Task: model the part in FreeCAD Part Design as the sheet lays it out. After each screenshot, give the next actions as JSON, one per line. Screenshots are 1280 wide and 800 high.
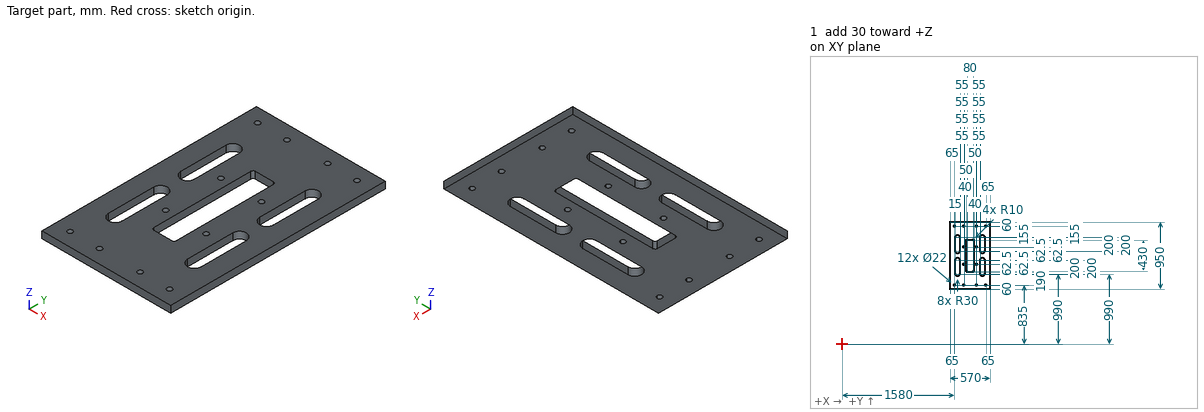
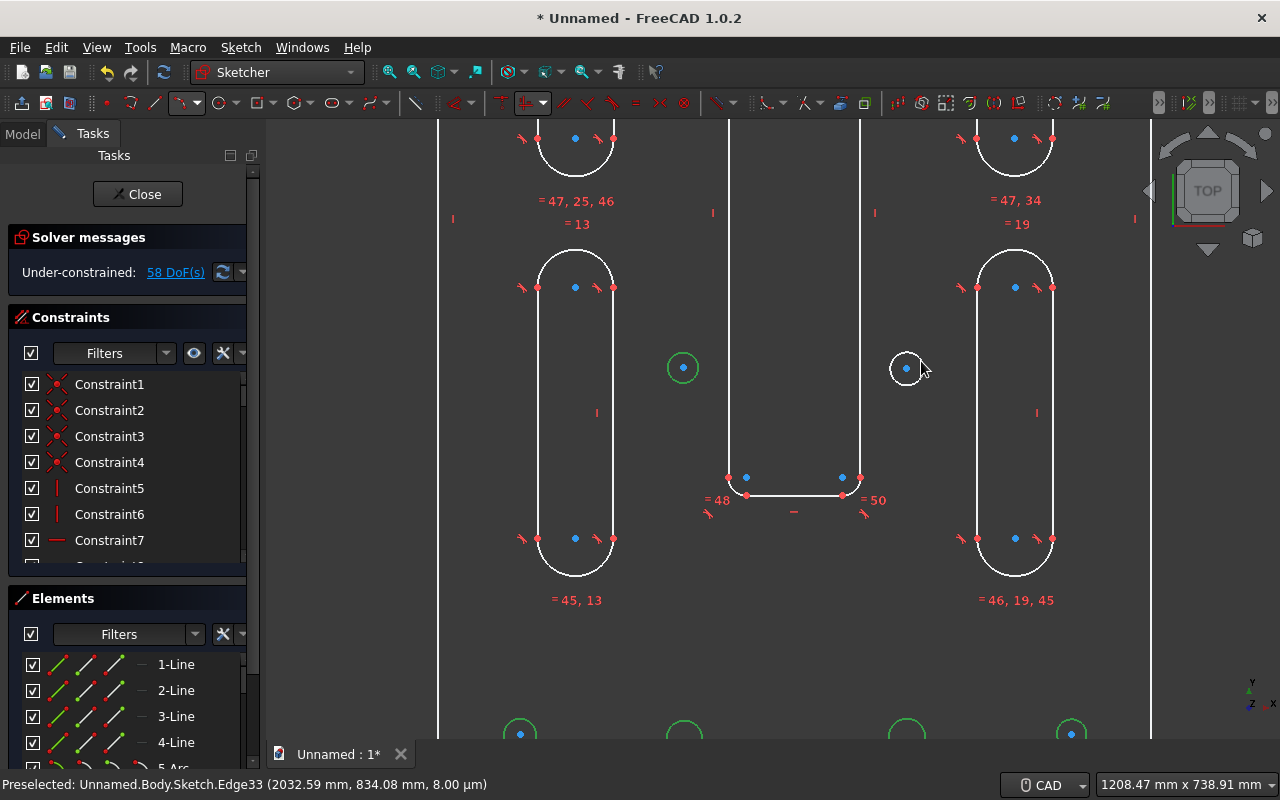
{"action": "left_click", "coordinate": [919, 357]}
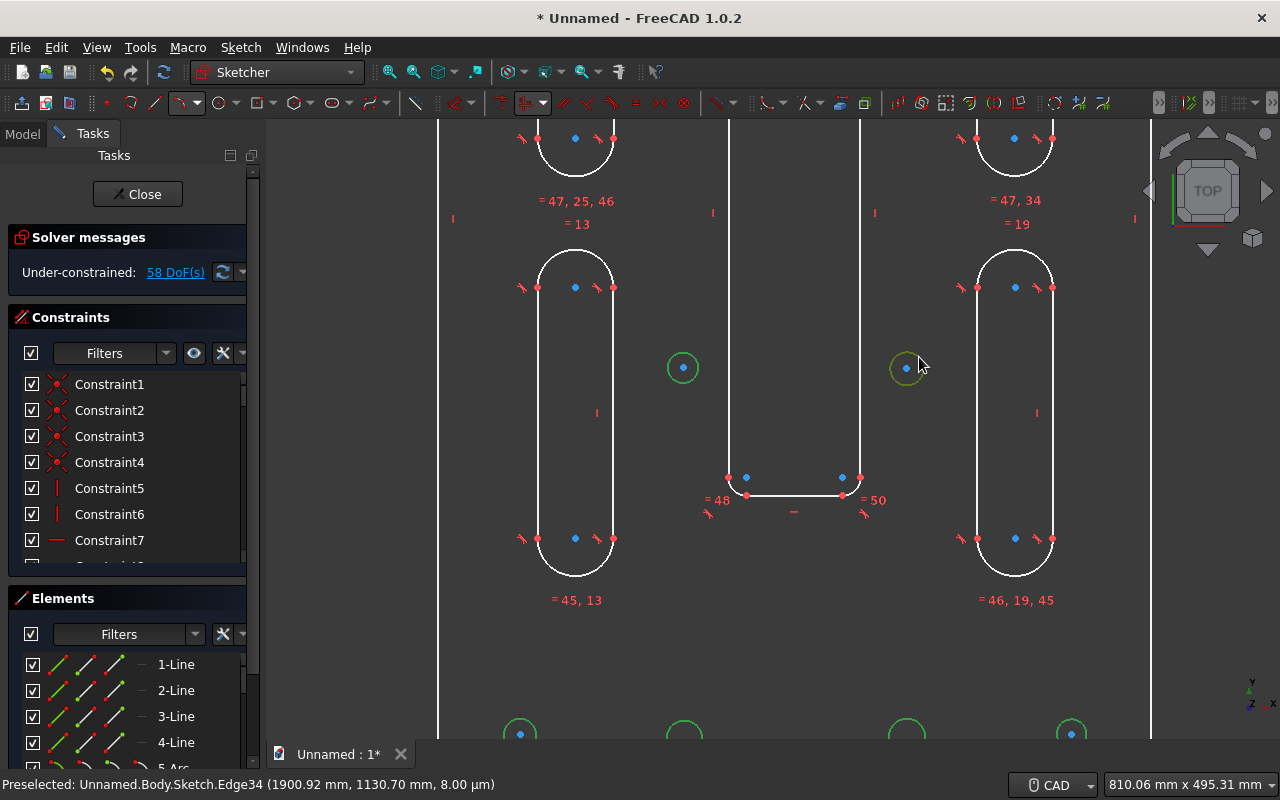
{"action": "scroll", "coordinate": [921, 361], "scroll_direction": "down", "scroll_amount": 8}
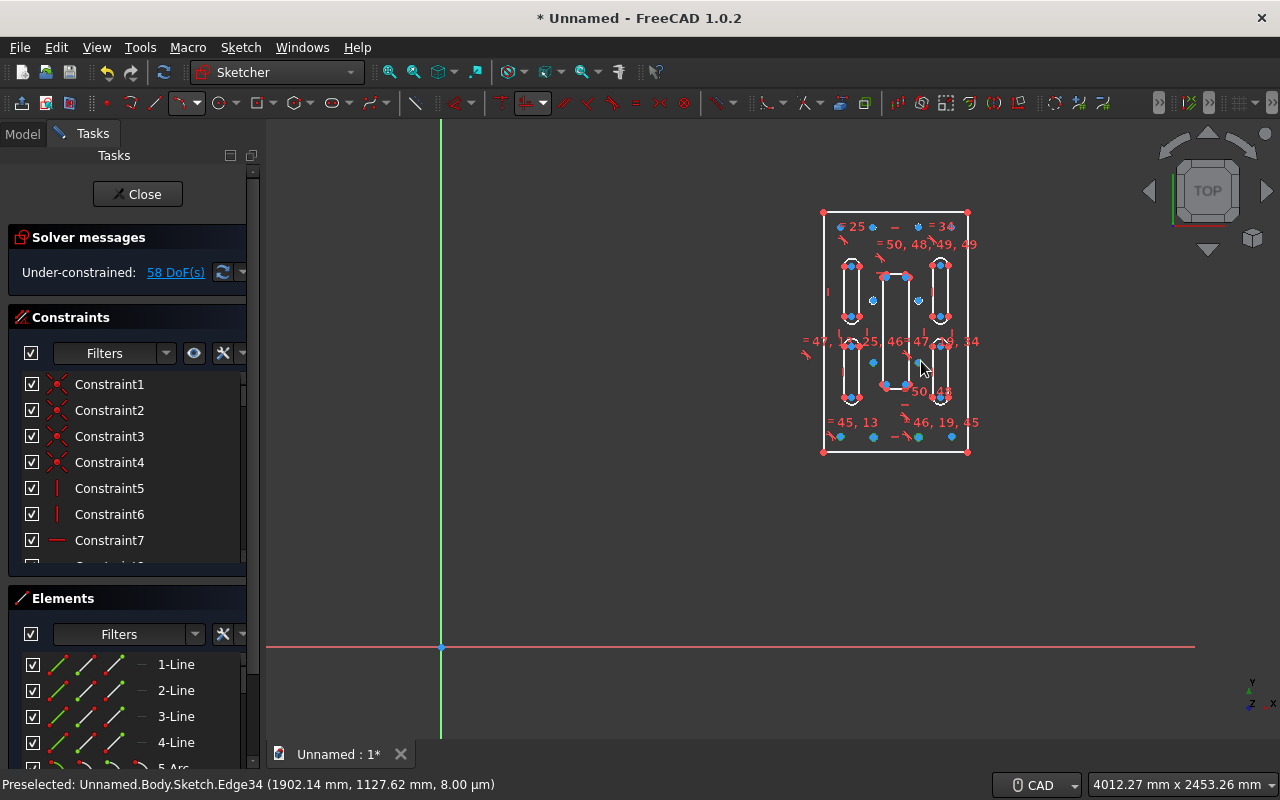
{"action": "scroll", "coordinate": [875, 298], "scroll_direction": "up", "scroll_amount": 8}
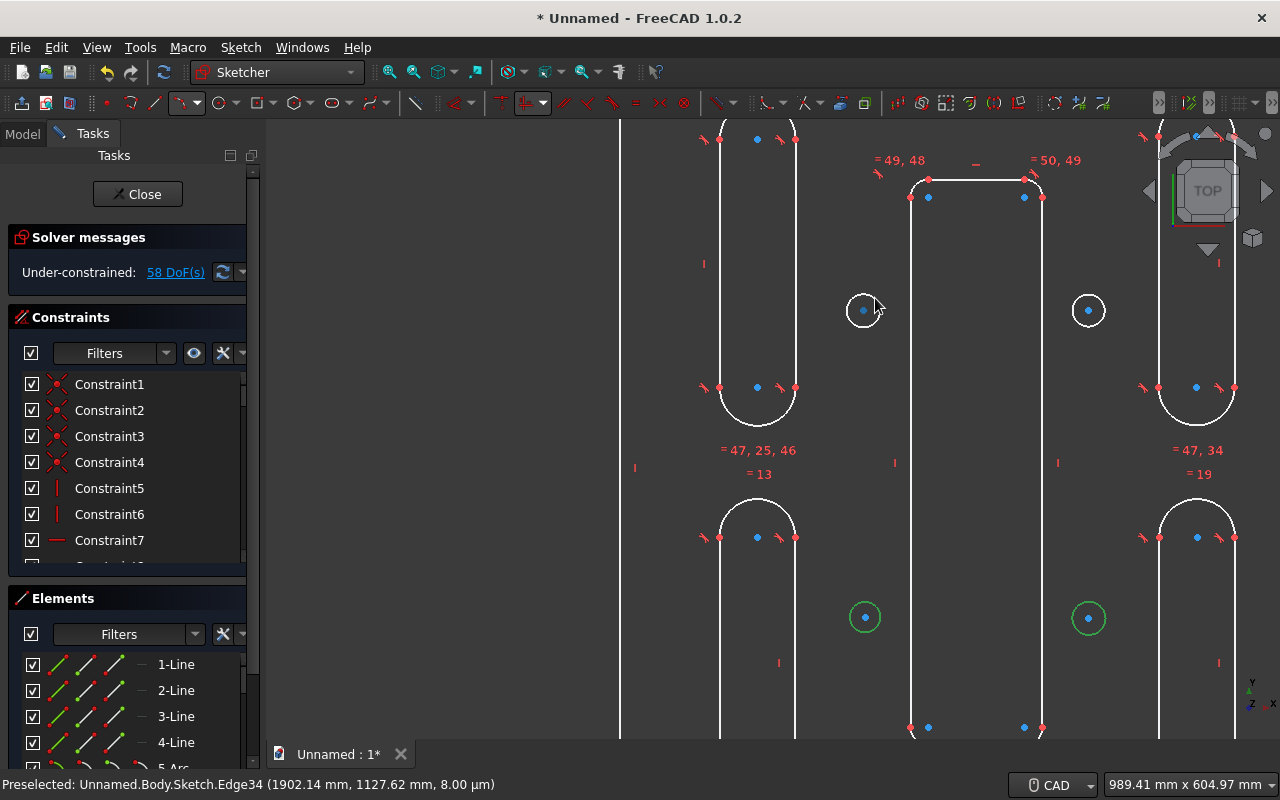
{"action": "left_click", "coordinate": [875, 299]}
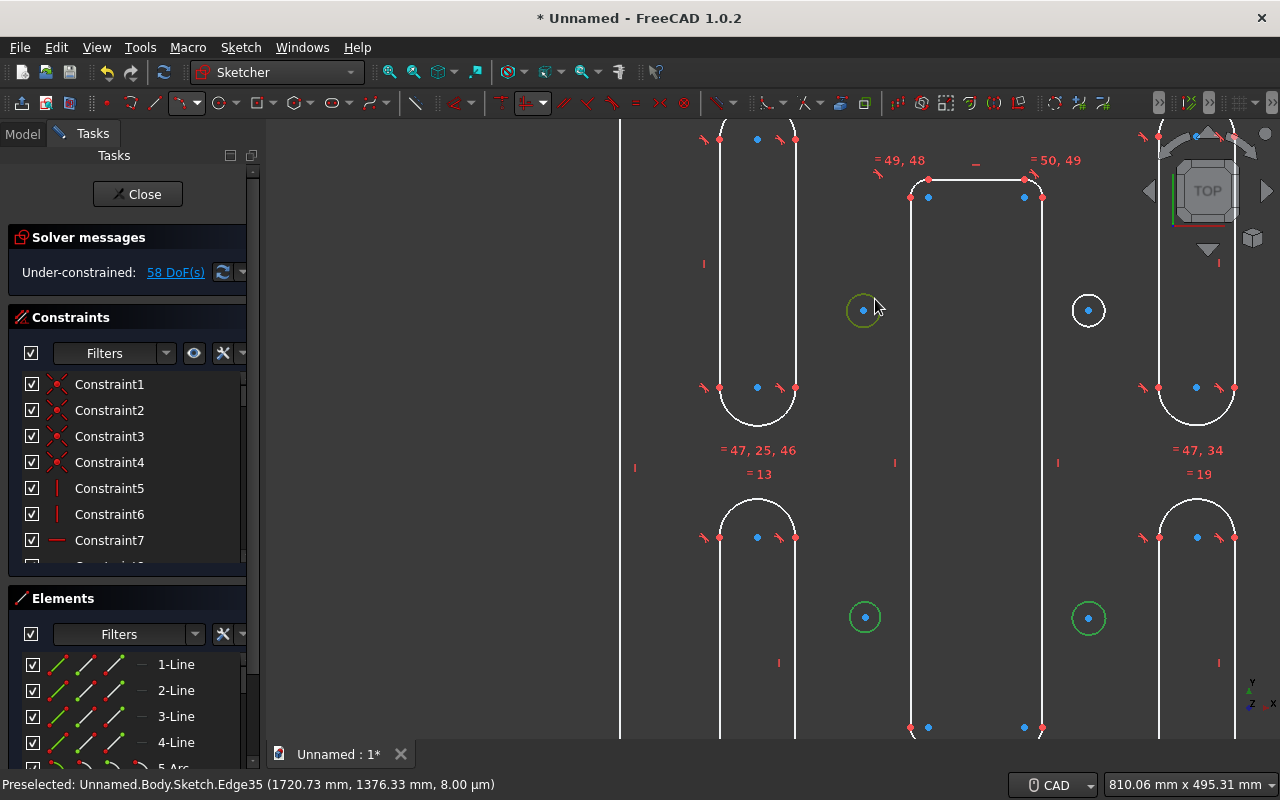
{"action": "scroll", "coordinate": [875, 298], "scroll_direction": "down", "scroll_amount": 8}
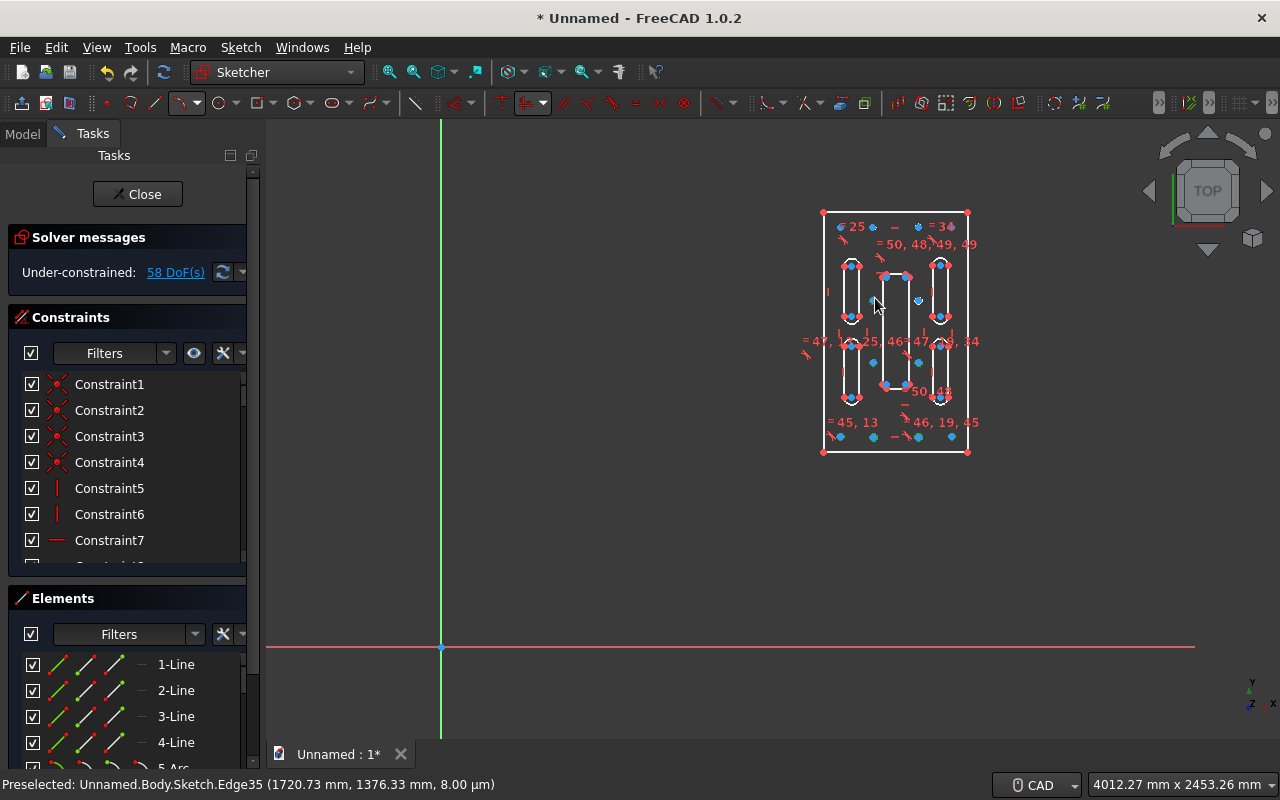
{"action": "scroll", "coordinate": [842, 226], "scroll_direction": "up", "scroll_amount": 10}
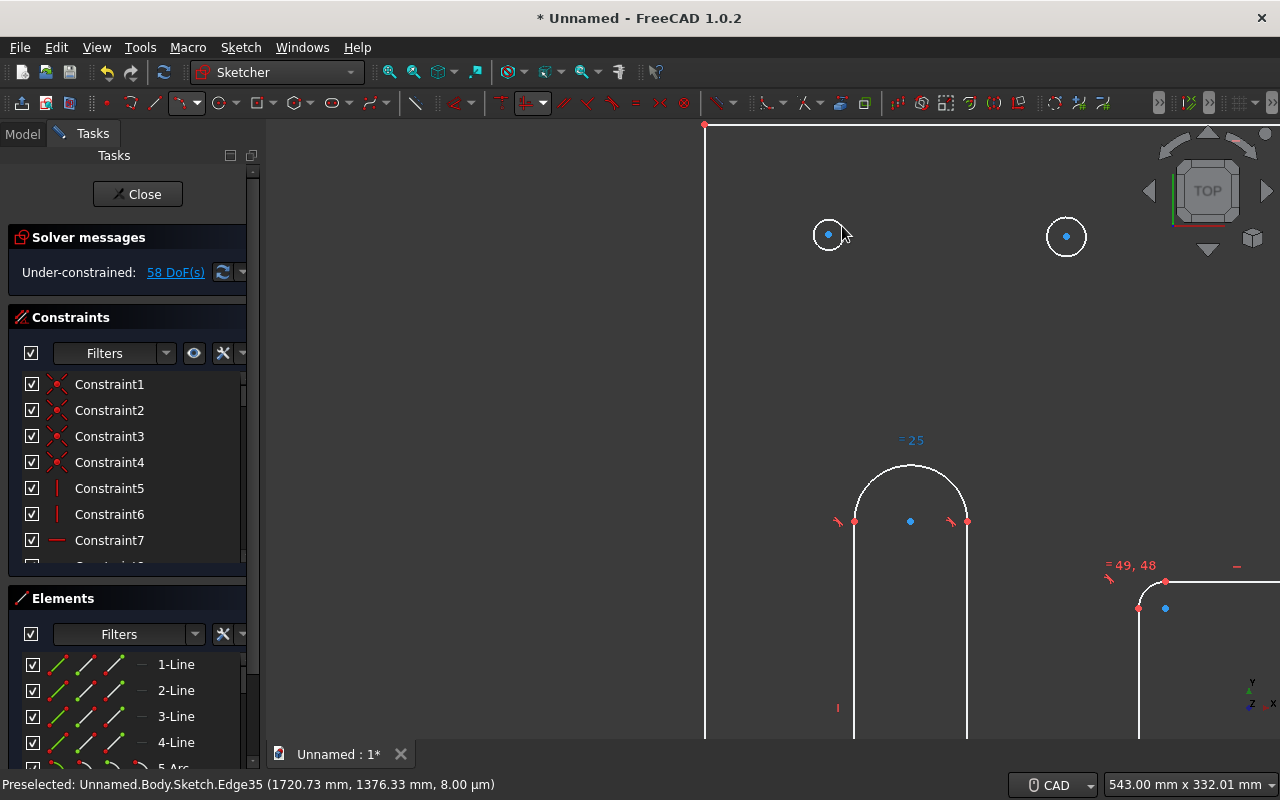
{"action": "left_click", "coordinate": [840, 224]}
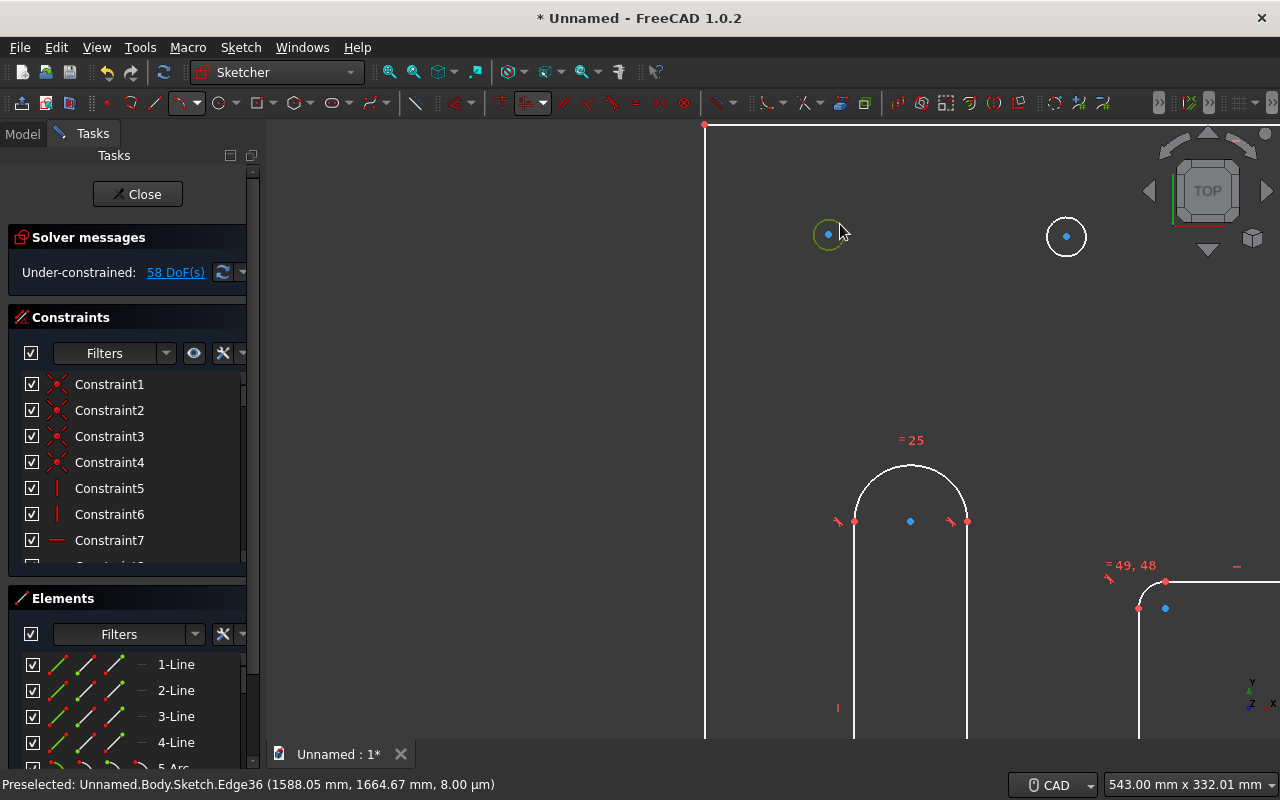
{"action": "left_click", "coordinate": [1080, 223]}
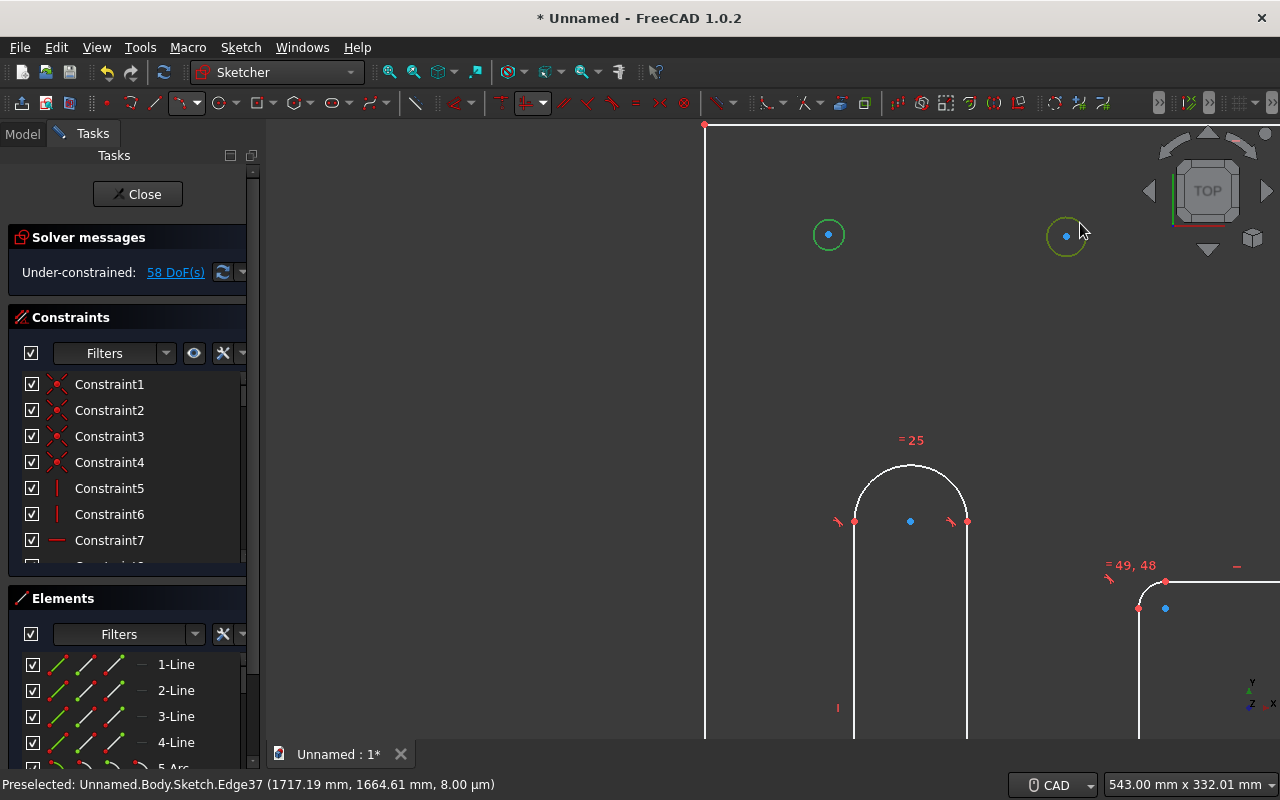
{"action": "scroll", "coordinate": [842, 226], "scroll_direction": "down", "scroll_amount": 10}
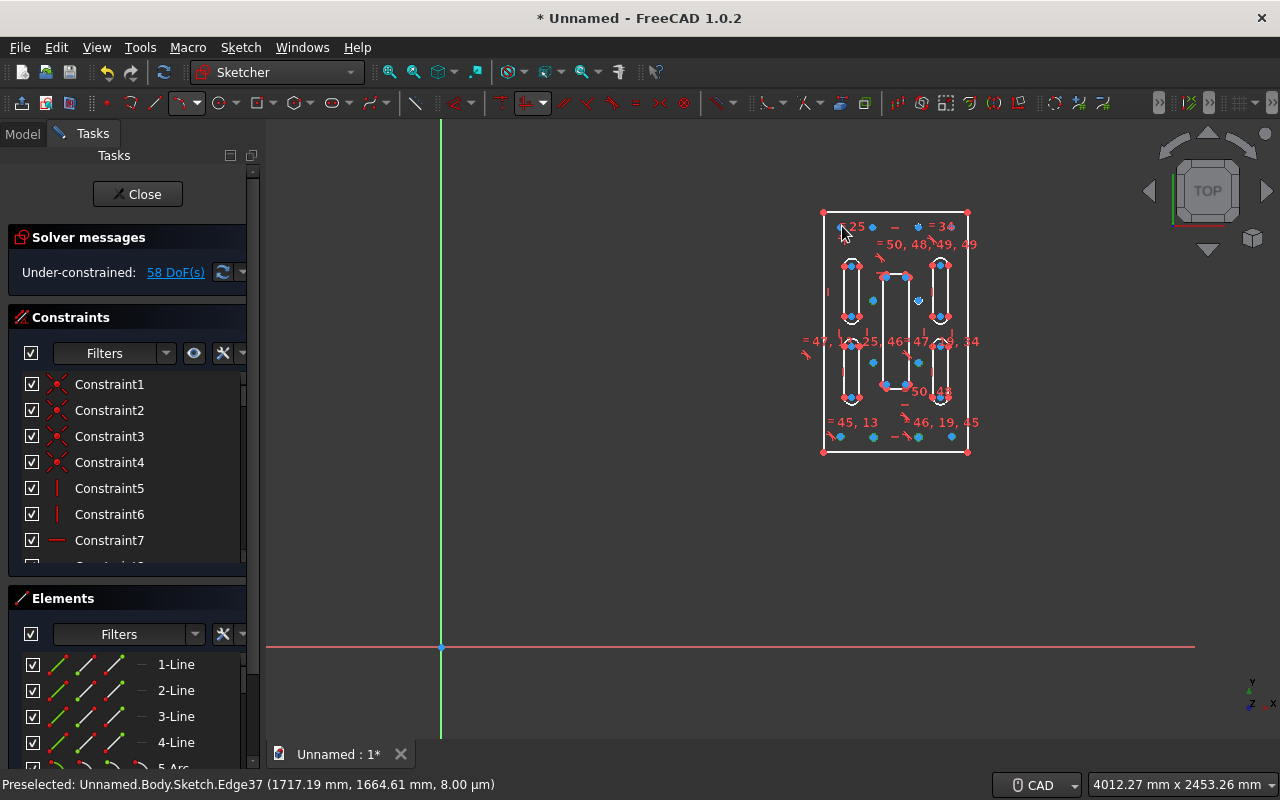
{"action": "scroll", "coordinate": [921, 298], "scroll_direction": "up", "scroll_amount": 8}